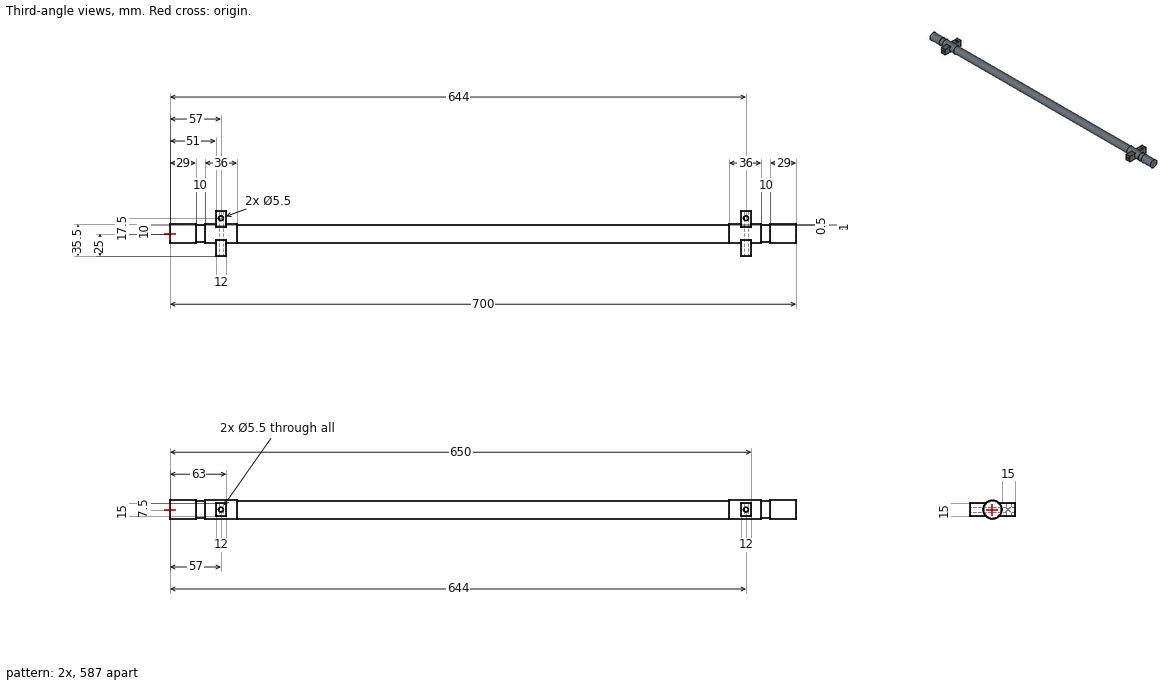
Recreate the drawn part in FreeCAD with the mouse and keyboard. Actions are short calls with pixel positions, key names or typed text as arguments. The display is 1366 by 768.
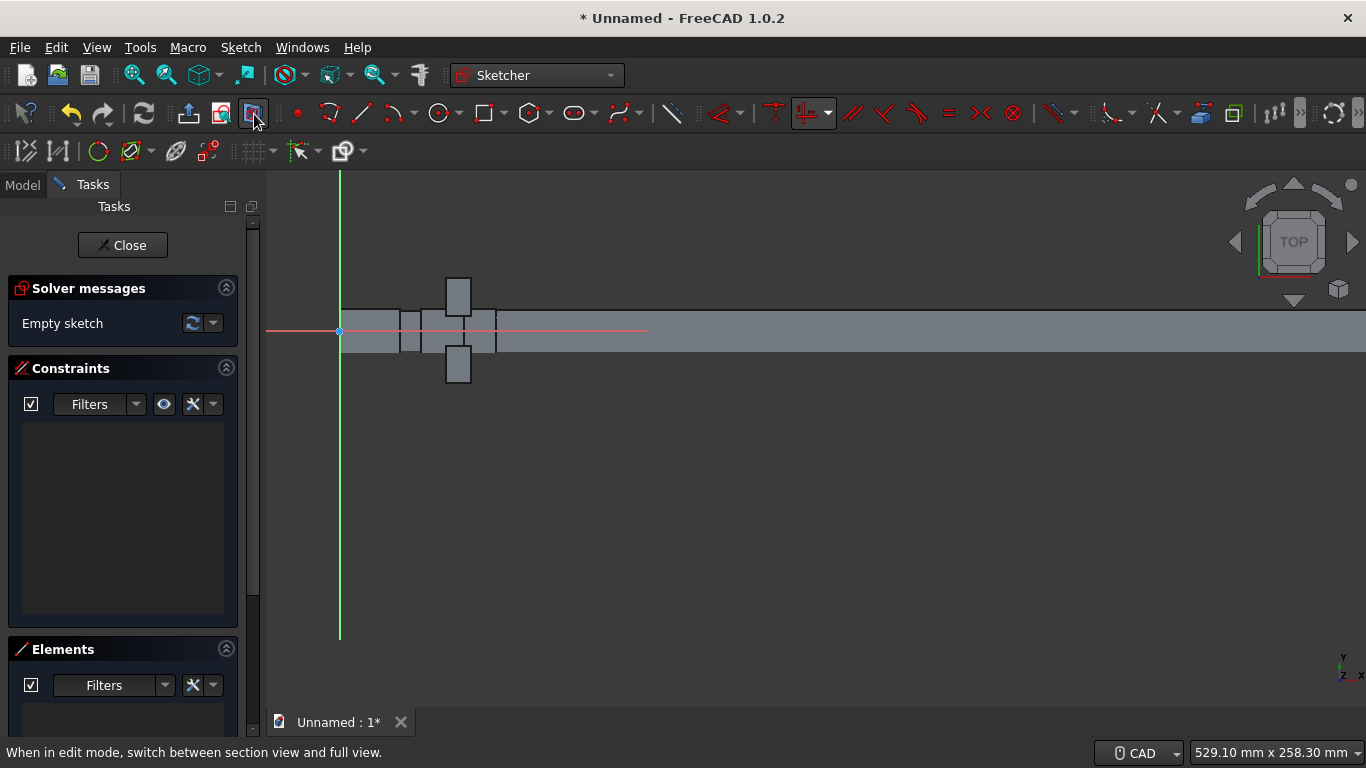
scroll(532, 543, down, 4)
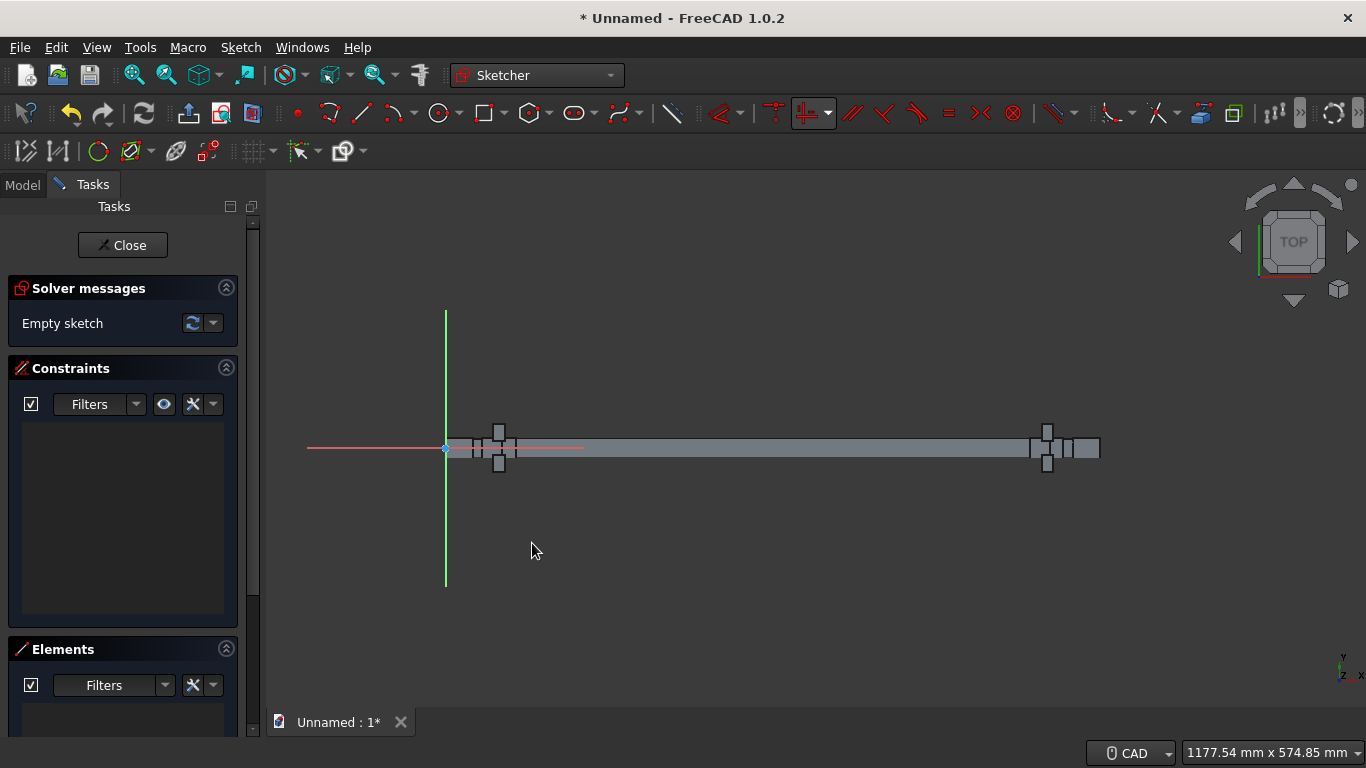
click(440, 114)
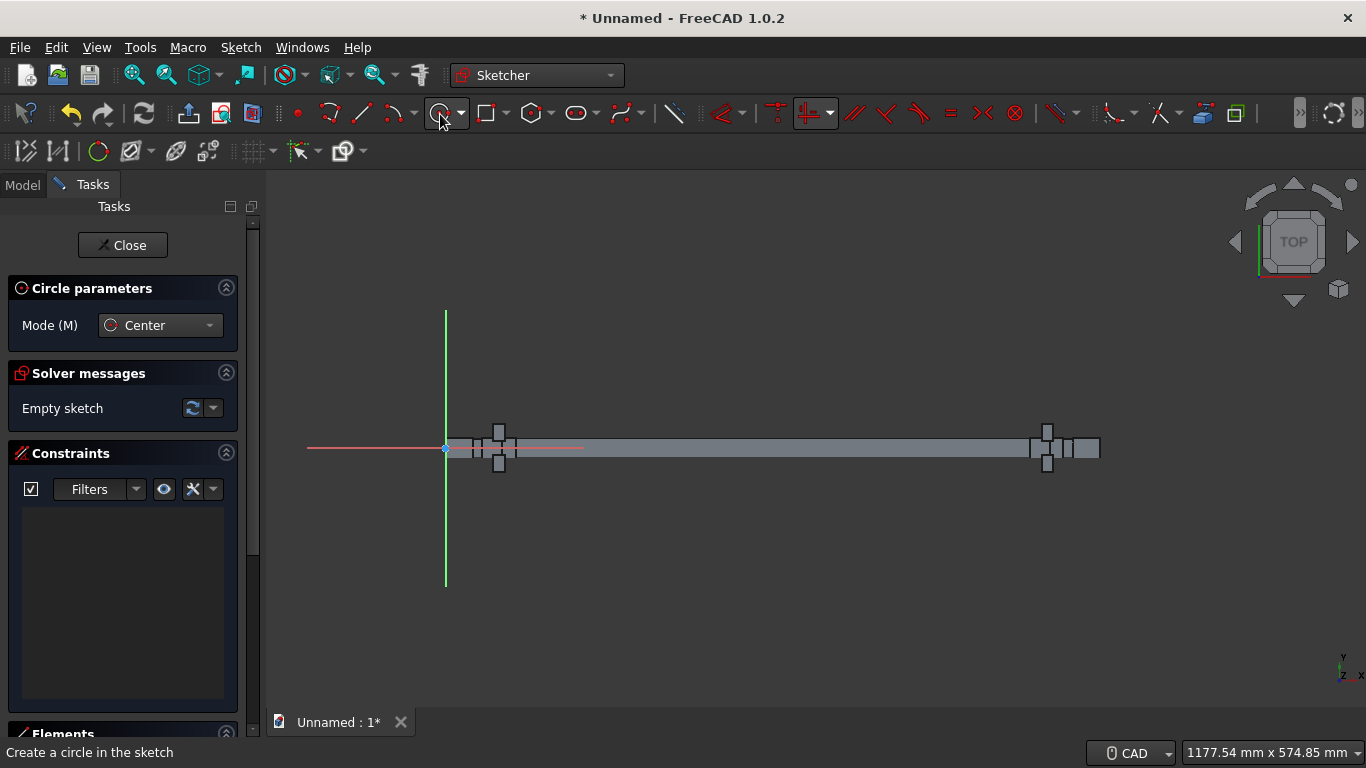
scroll(499, 432, up, 11)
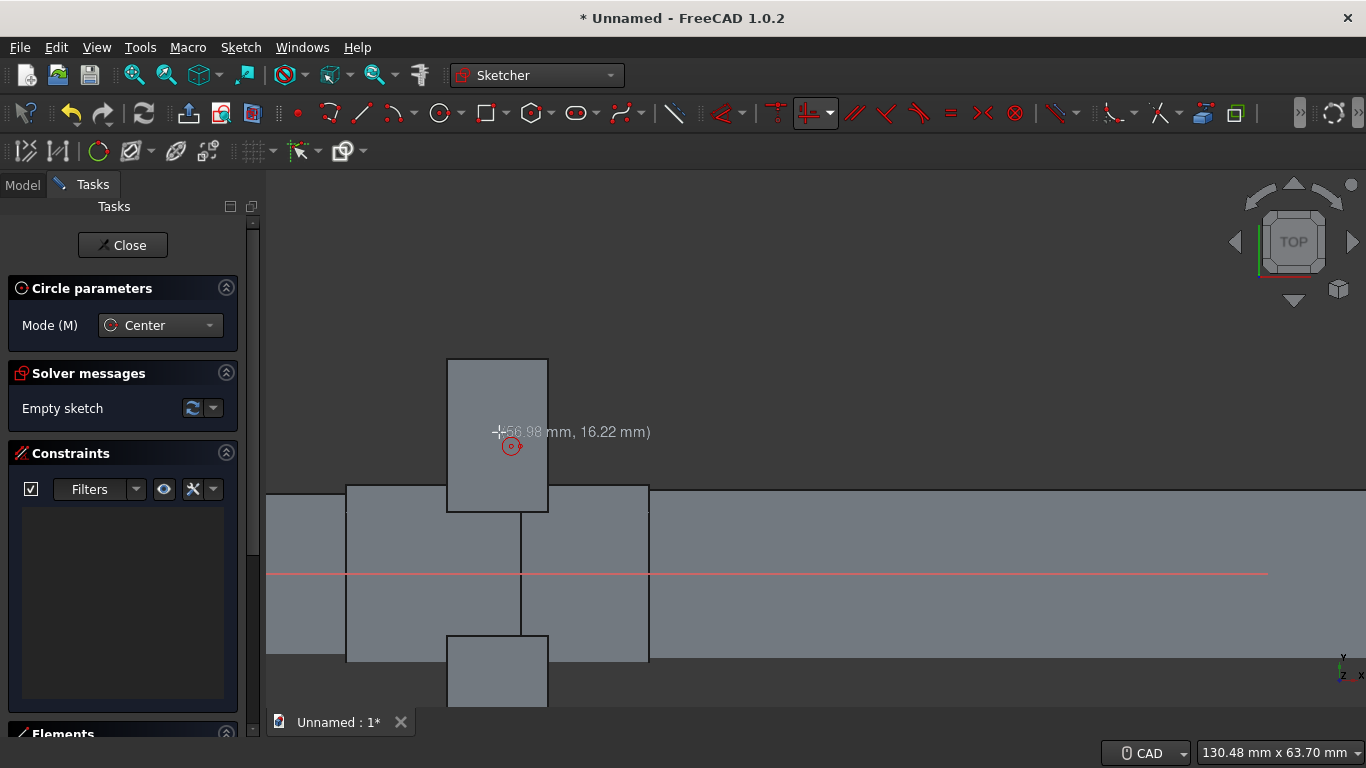
scroll(499, 432, down, 11)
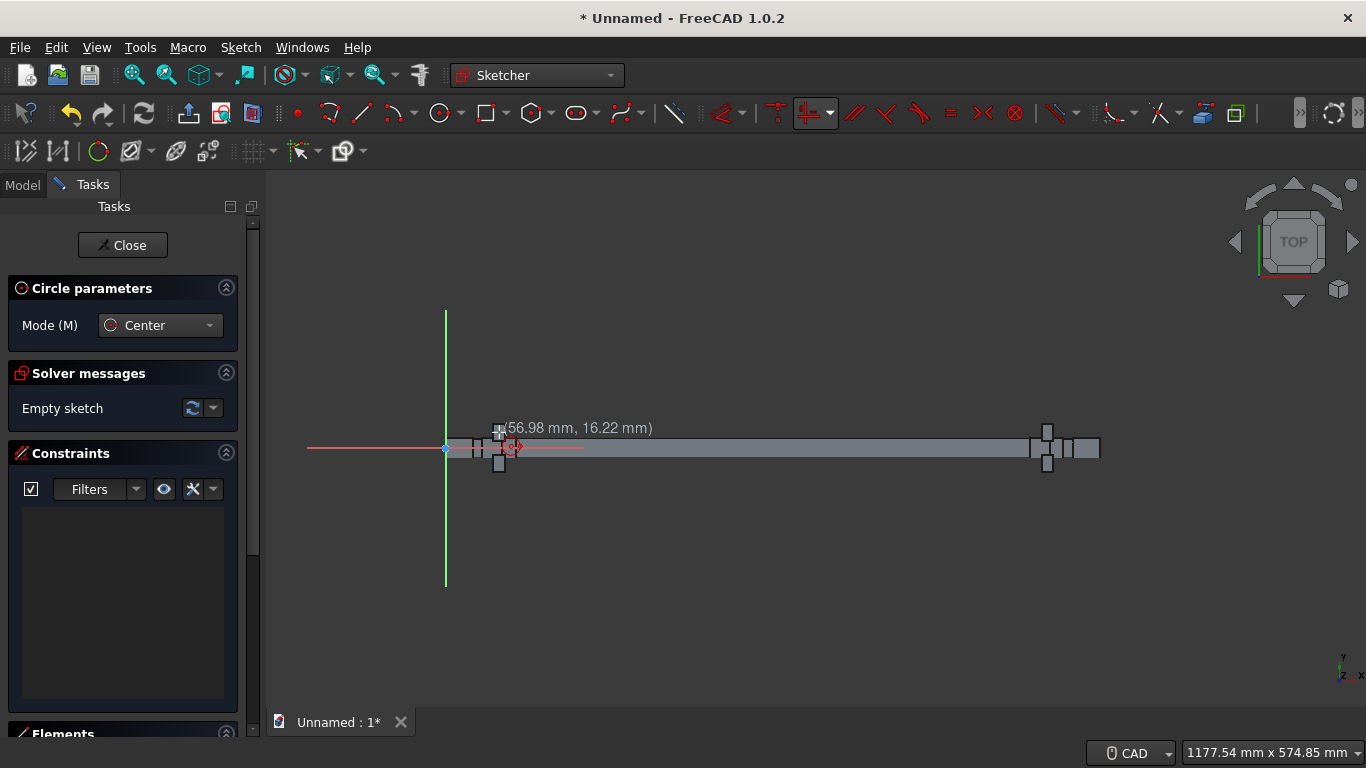
click(499, 432)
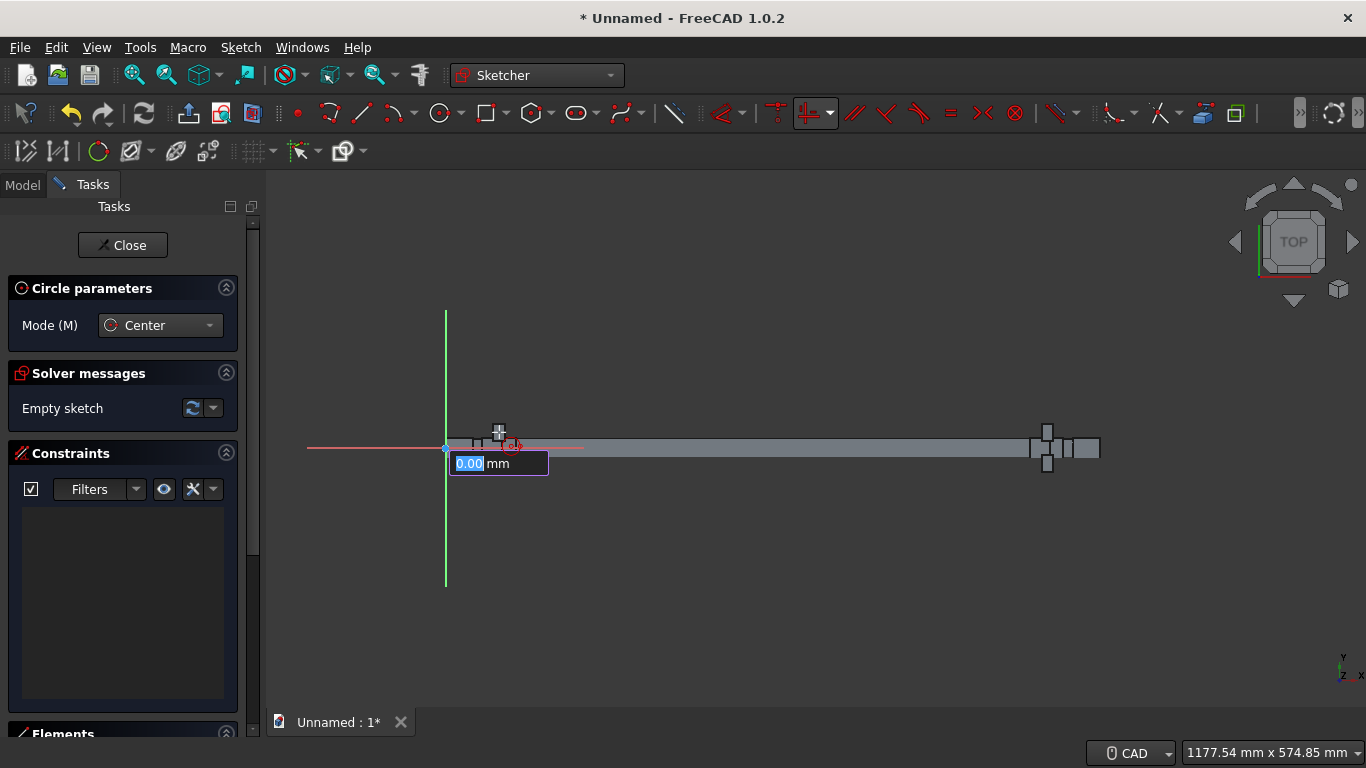
scroll(501, 430, up, 10)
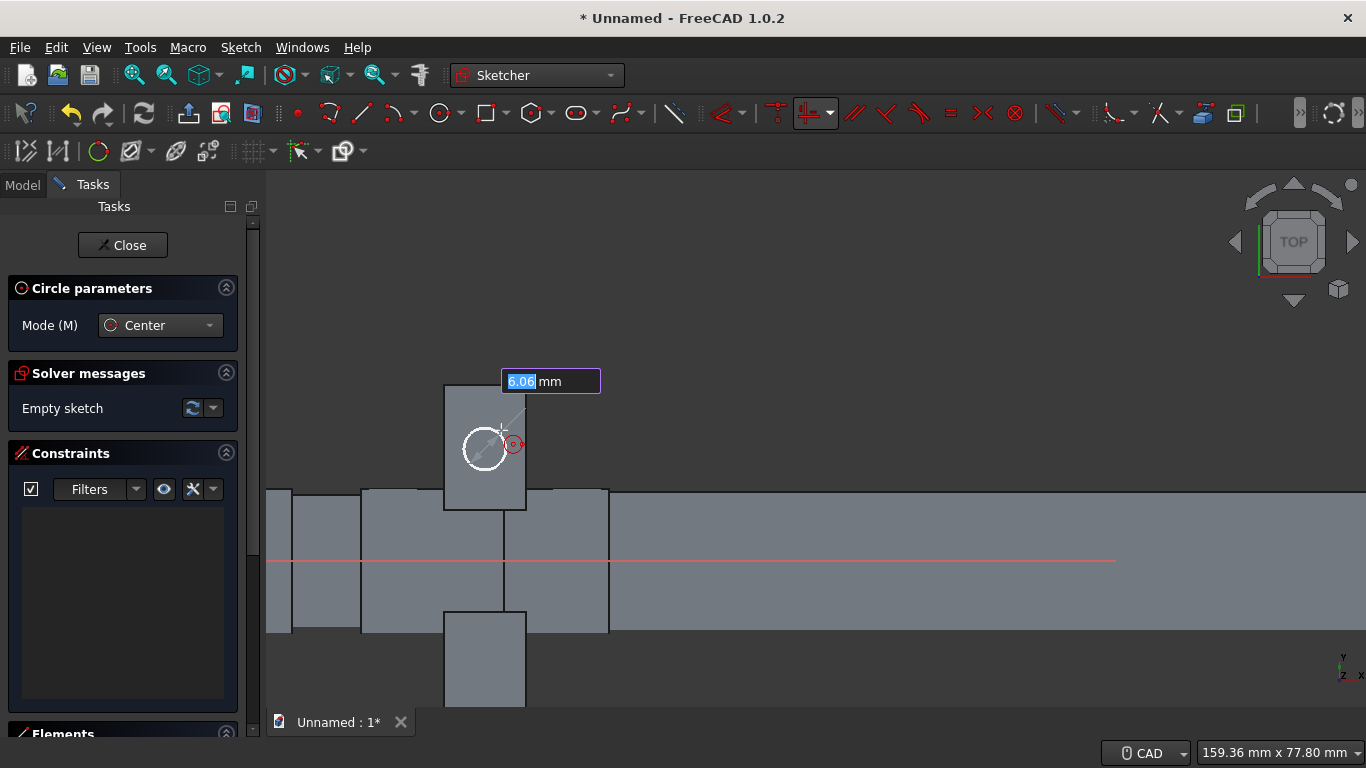
click(498, 427)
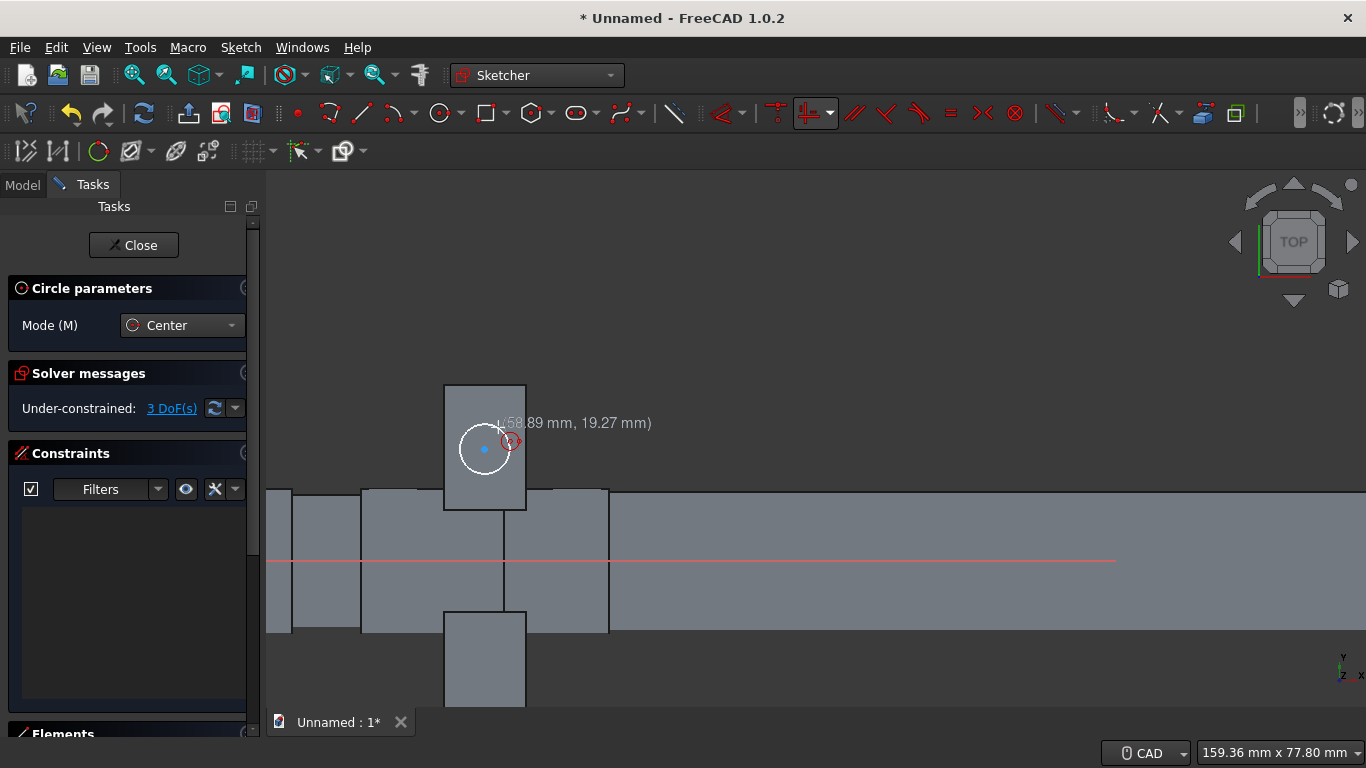
scroll(501, 430, down, 10)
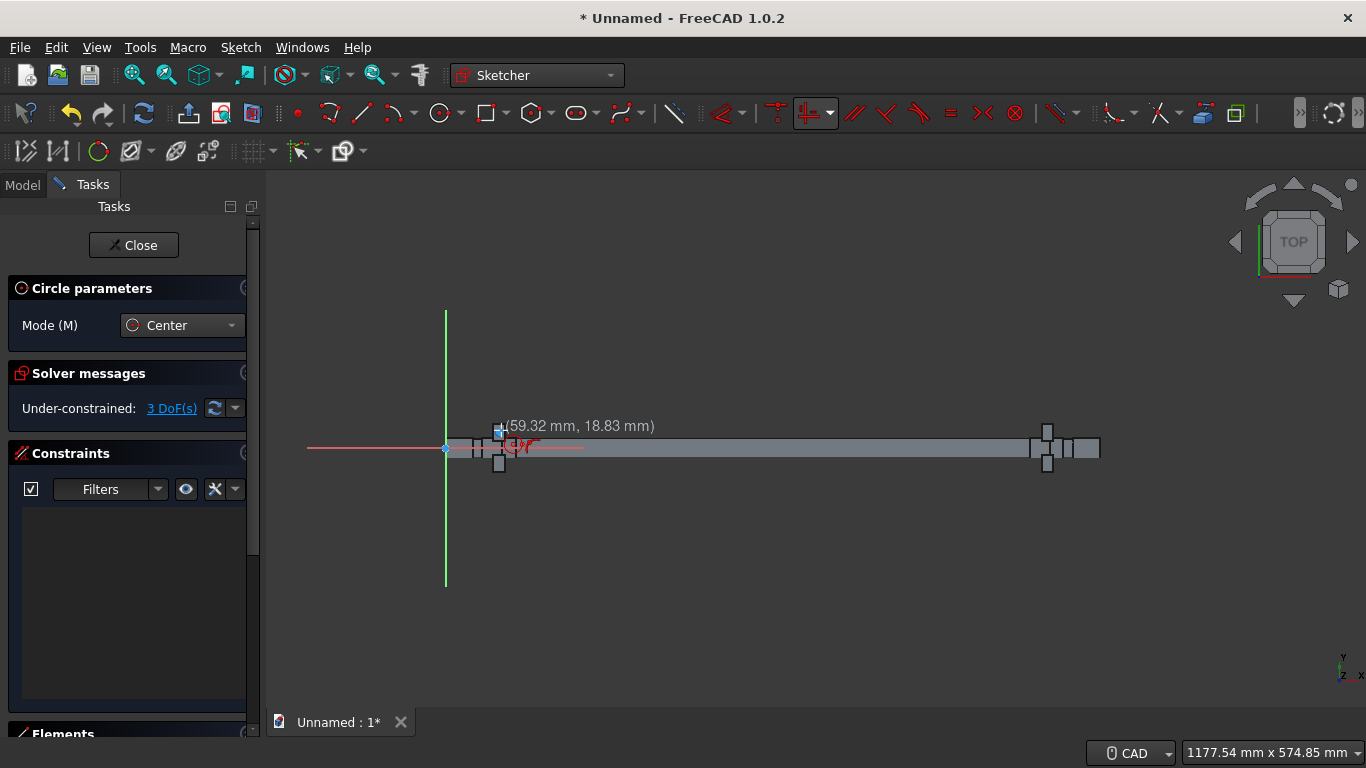
scroll(1047, 432, up, 11)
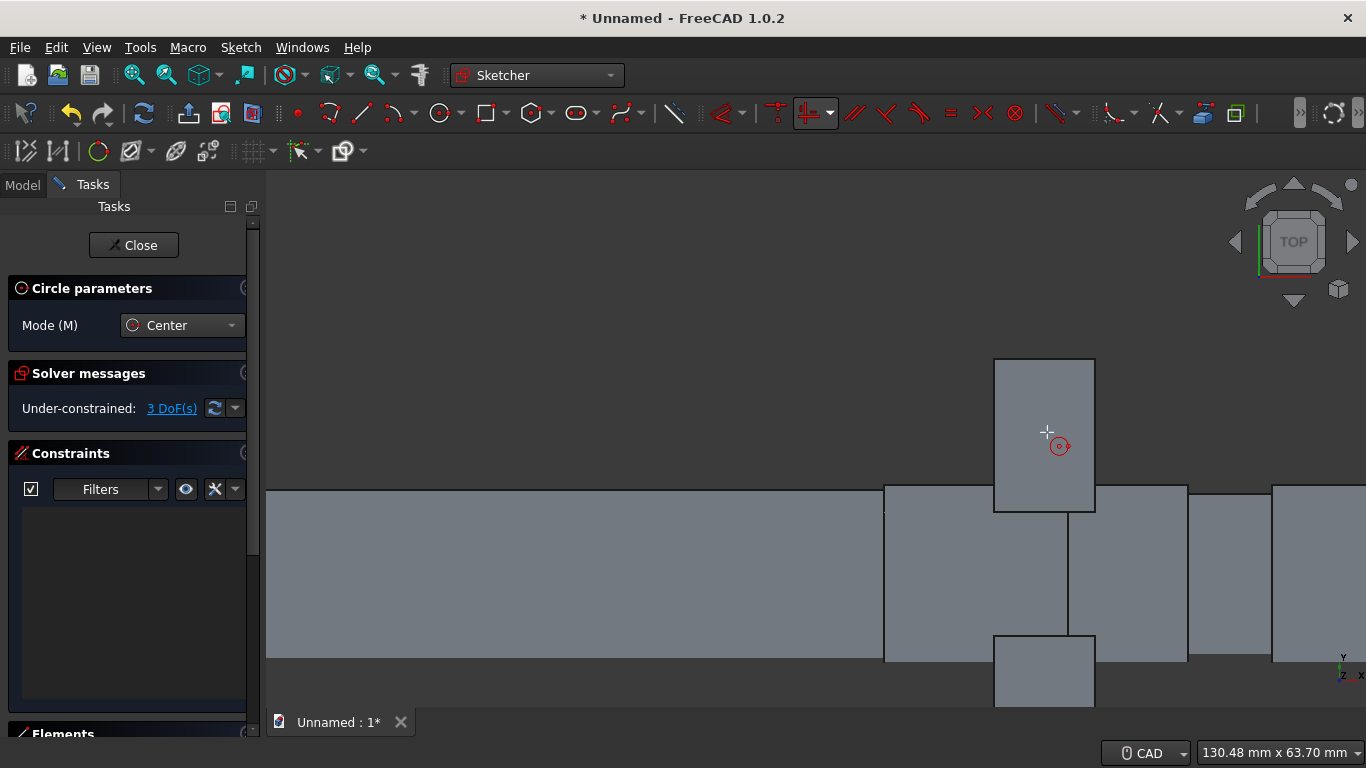
scroll(1047, 432, down, 11)